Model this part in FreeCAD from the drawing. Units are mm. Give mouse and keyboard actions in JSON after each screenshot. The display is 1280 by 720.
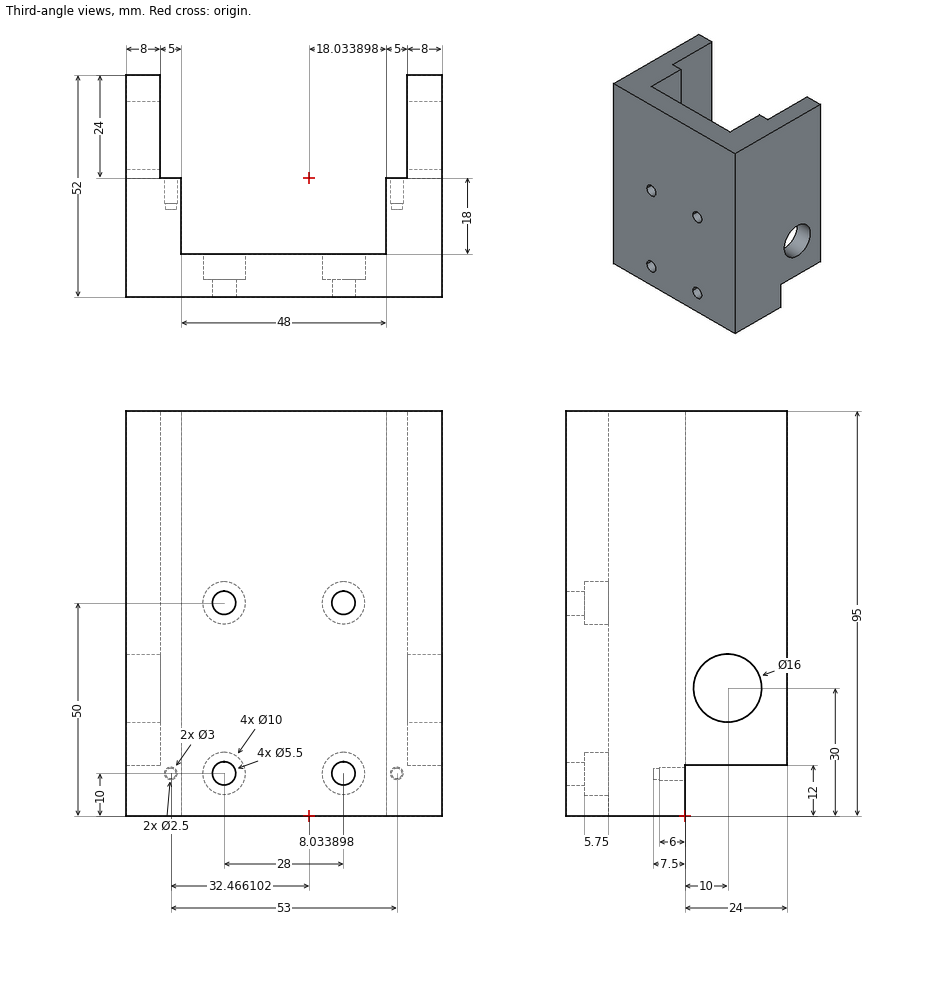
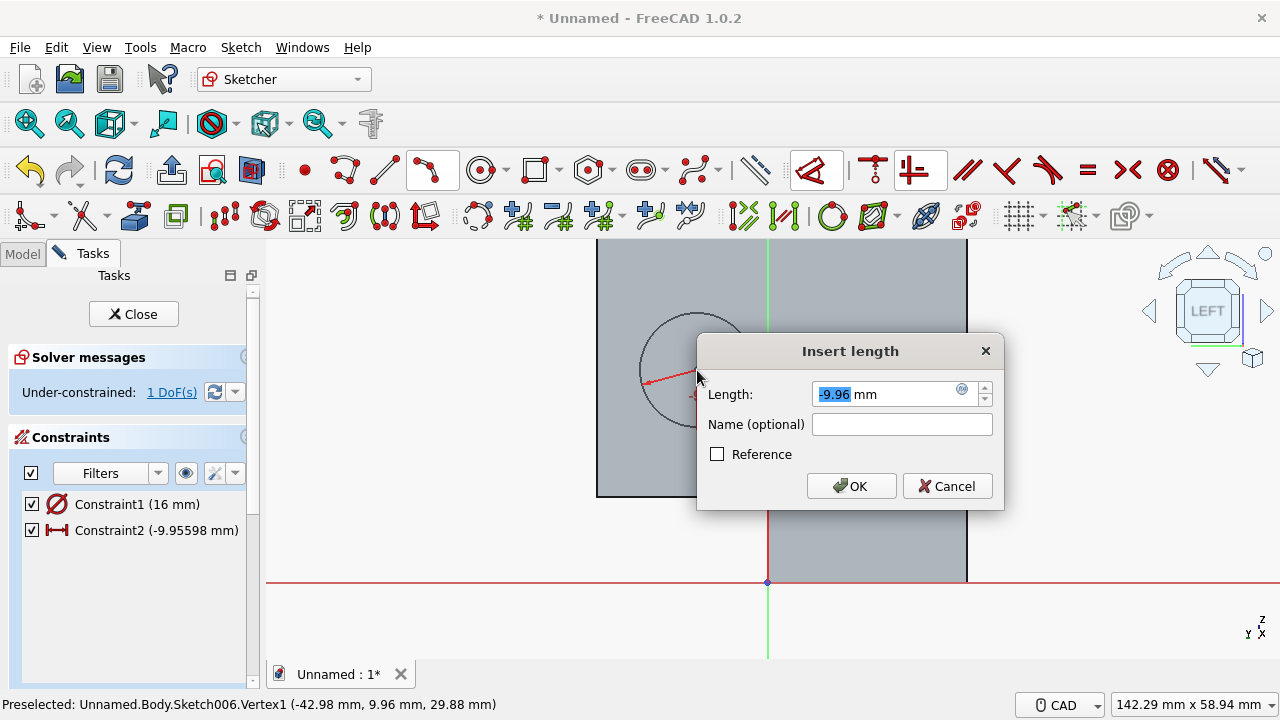
{"action": "type", "text": "-10"}
{"action": "key", "text": "Return"}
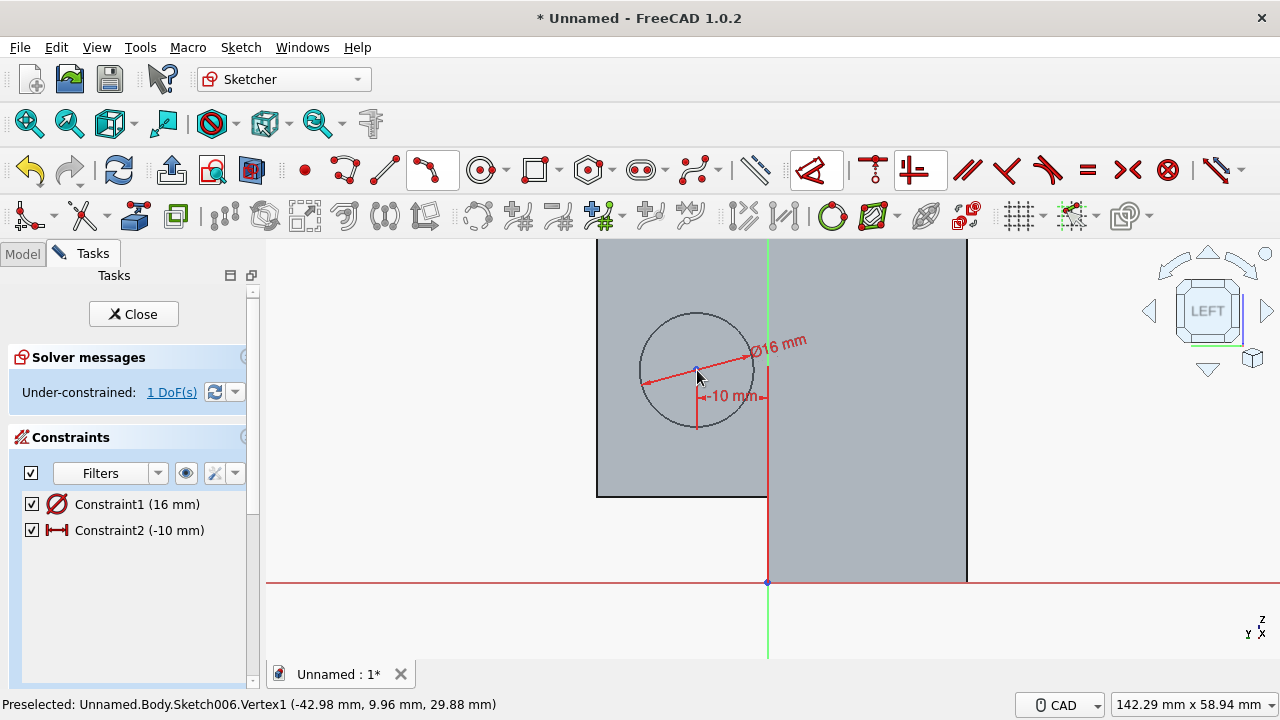
{"action": "left_click", "coordinate": [697, 370]}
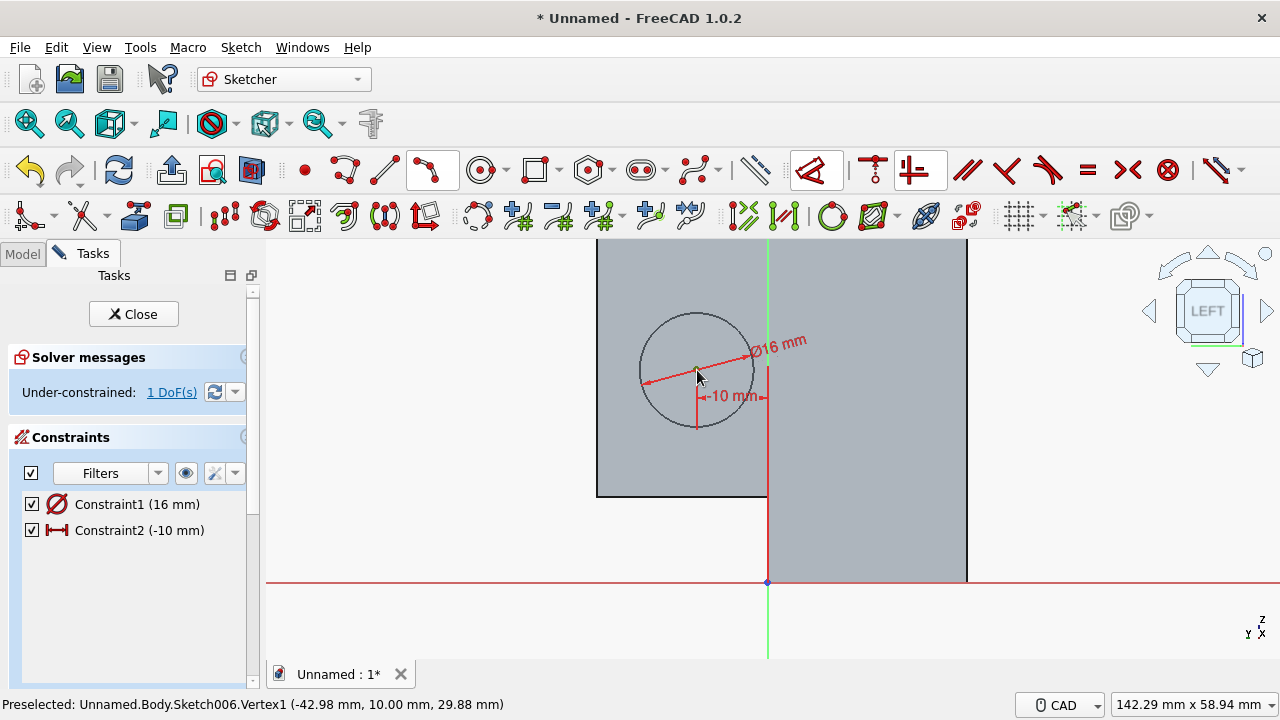
{"action": "key", "text": "i"}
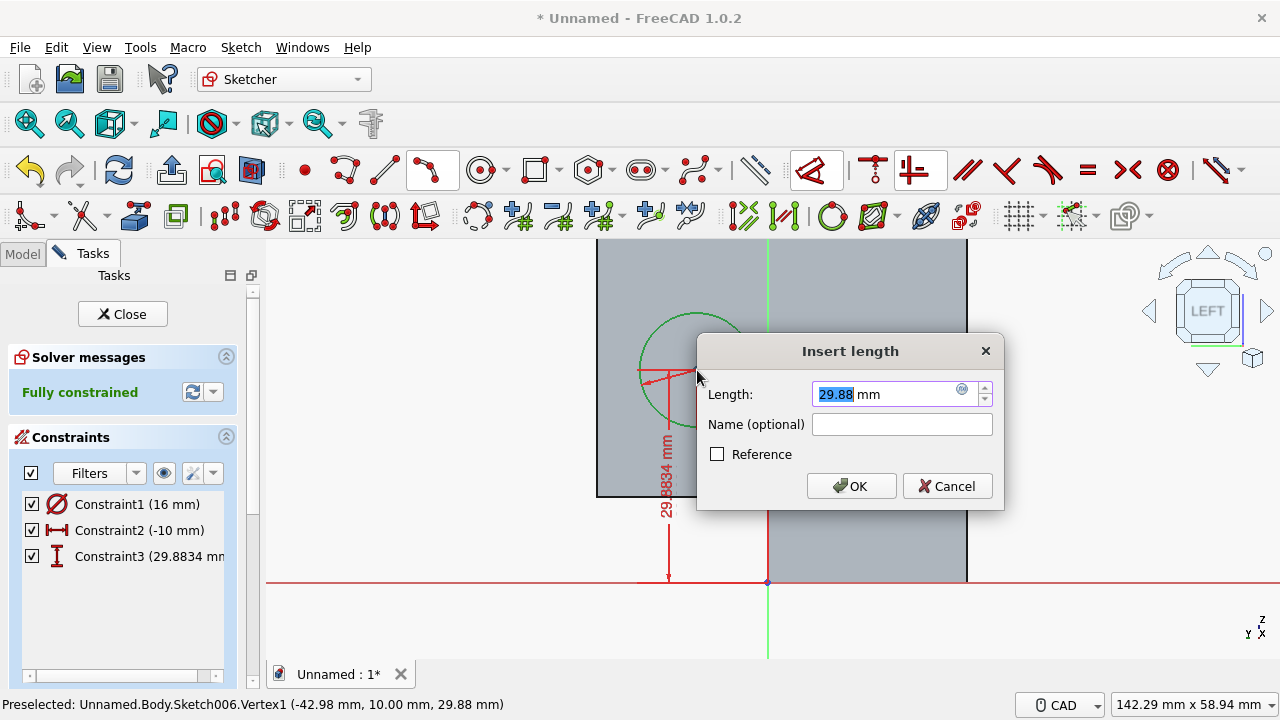
{"action": "type", "text": "30"}
{"action": "key", "text": "Return"}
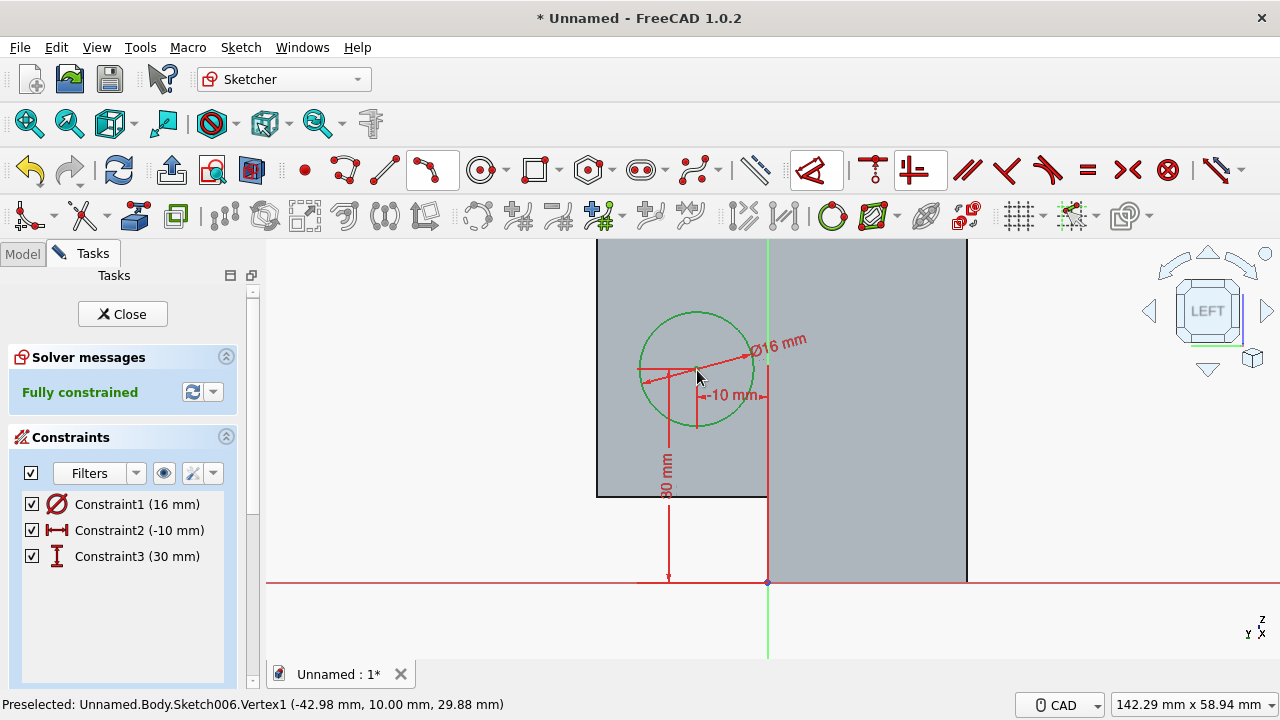
{"action": "left_click", "coordinate": [123, 314]}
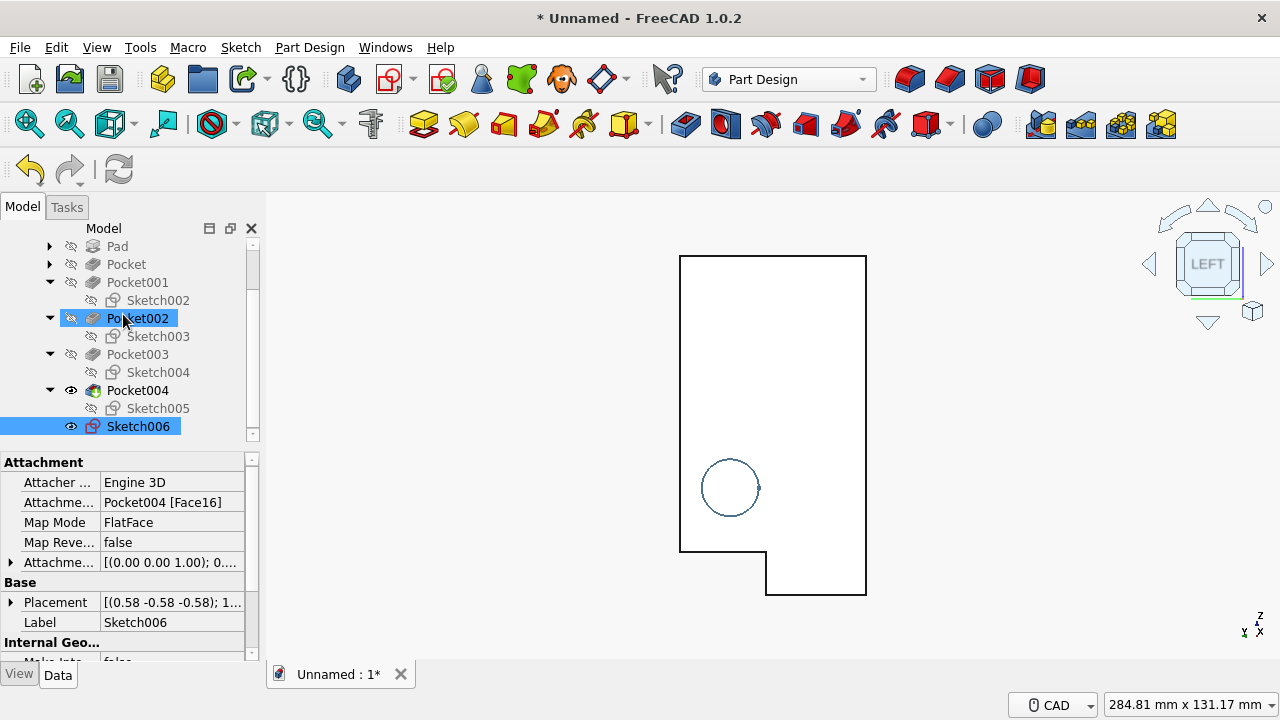
{"action": "left_click", "coordinate": [686, 124]}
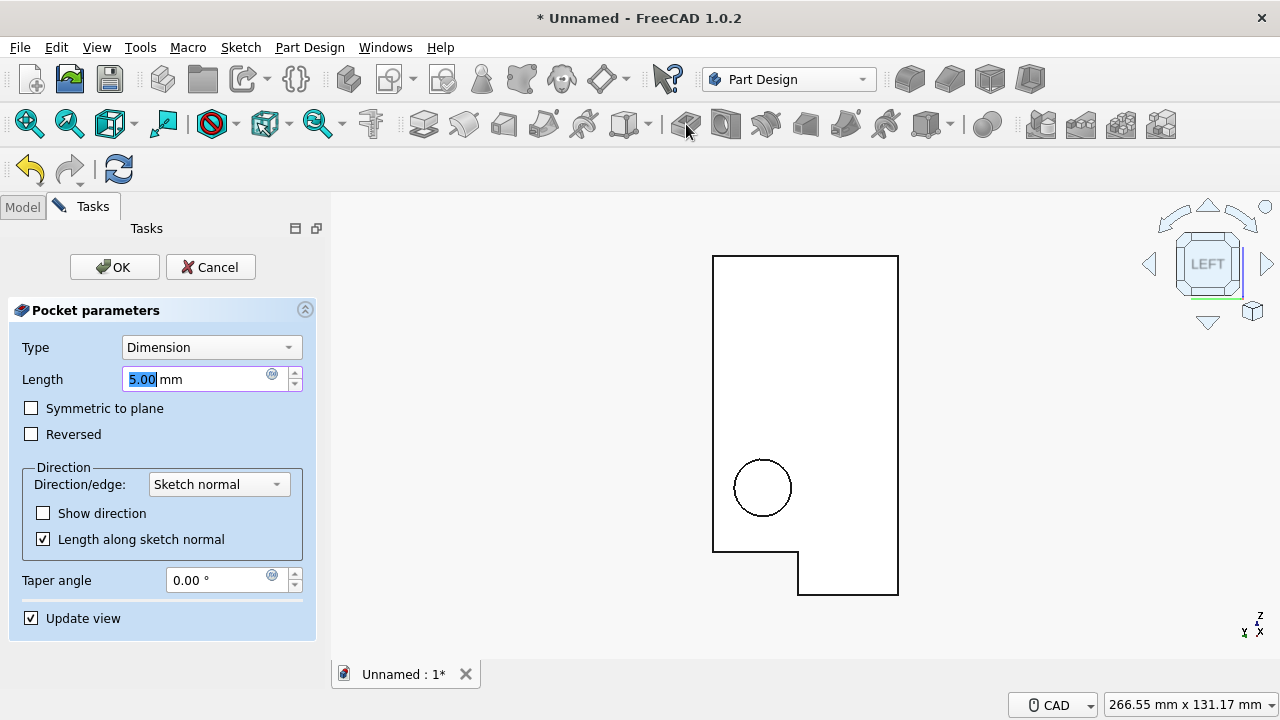
{"action": "left_click", "coordinate": [212, 348]}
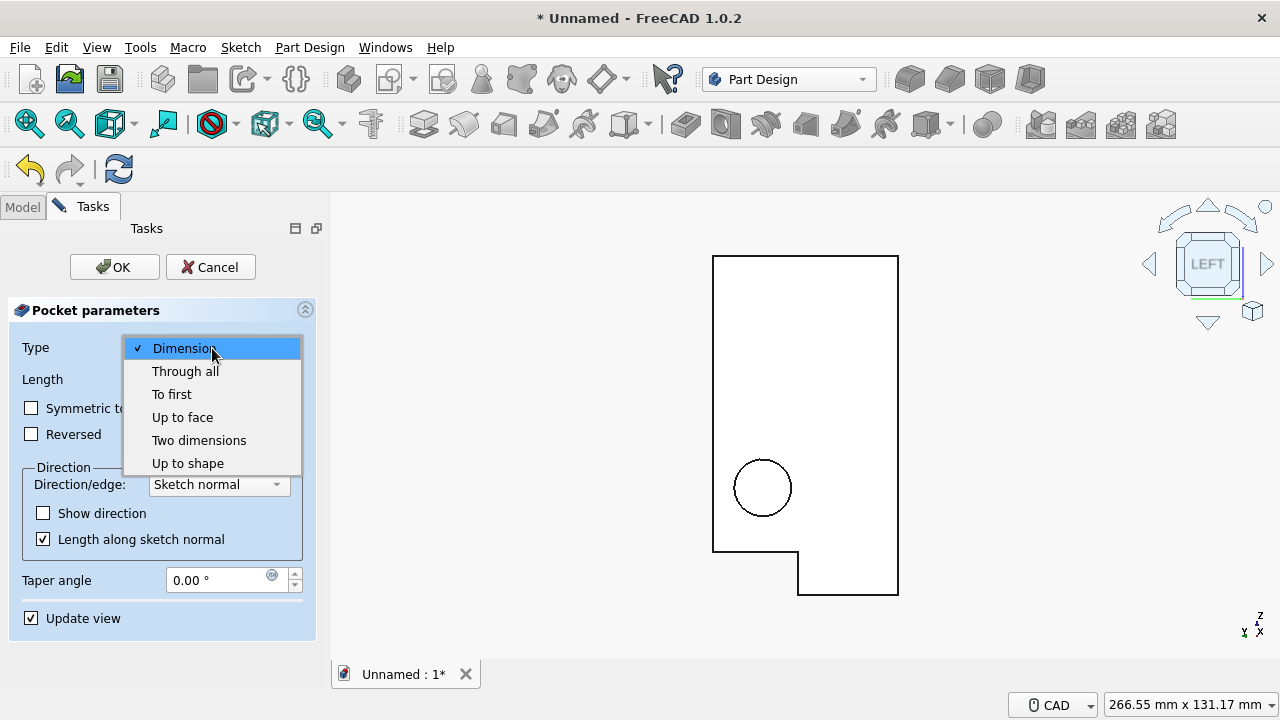
{"action": "left_click", "coordinate": [212, 372]}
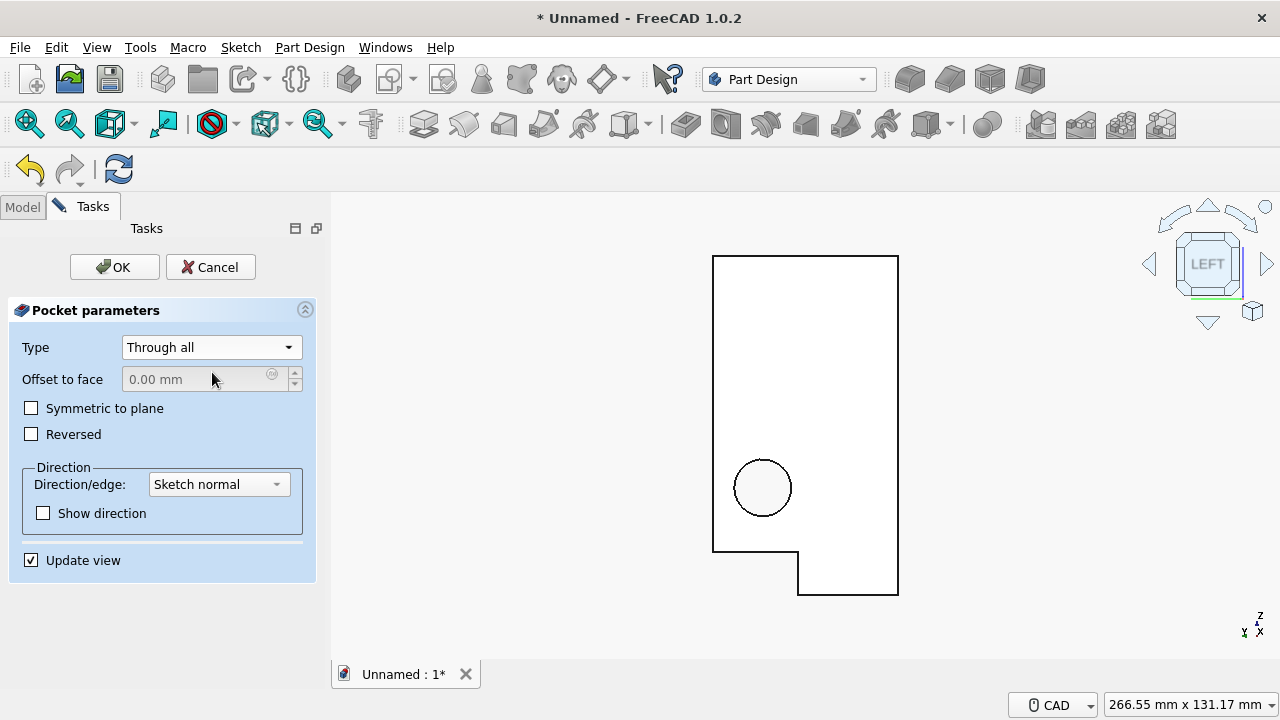
{"action": "left_click", "coordinate": [115, 267]}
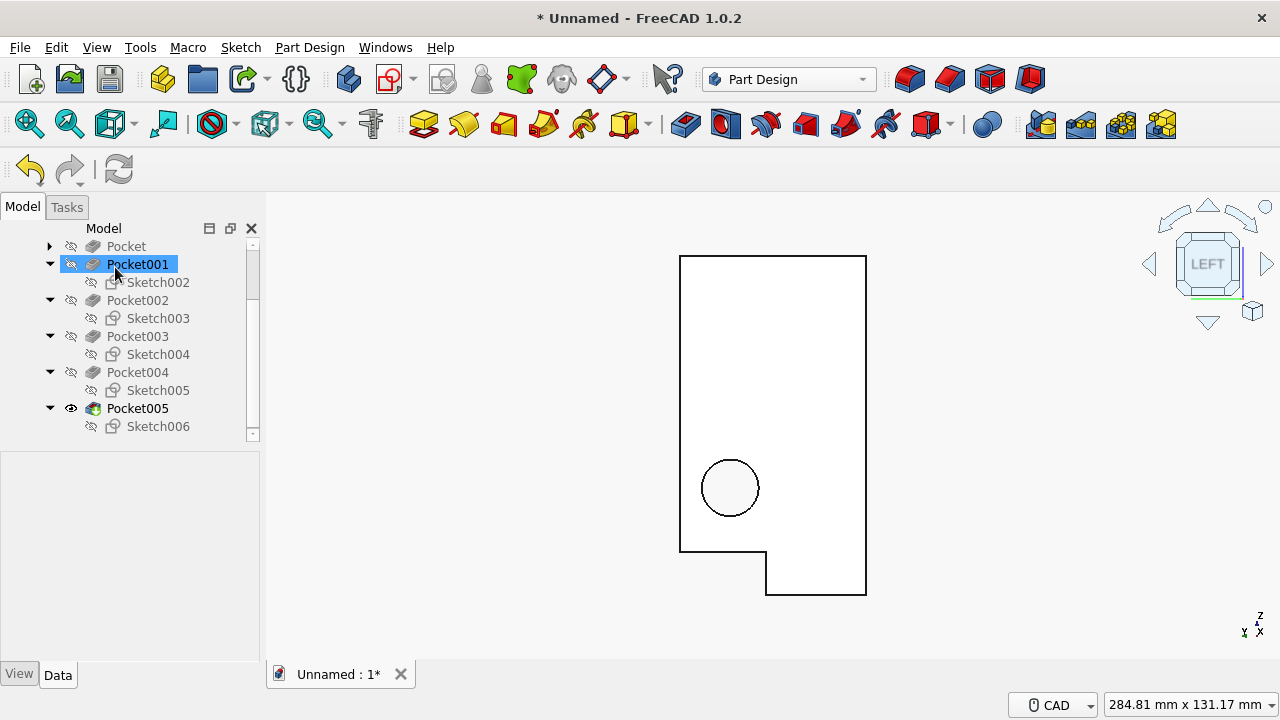
{"action": "key", "text": "0"}